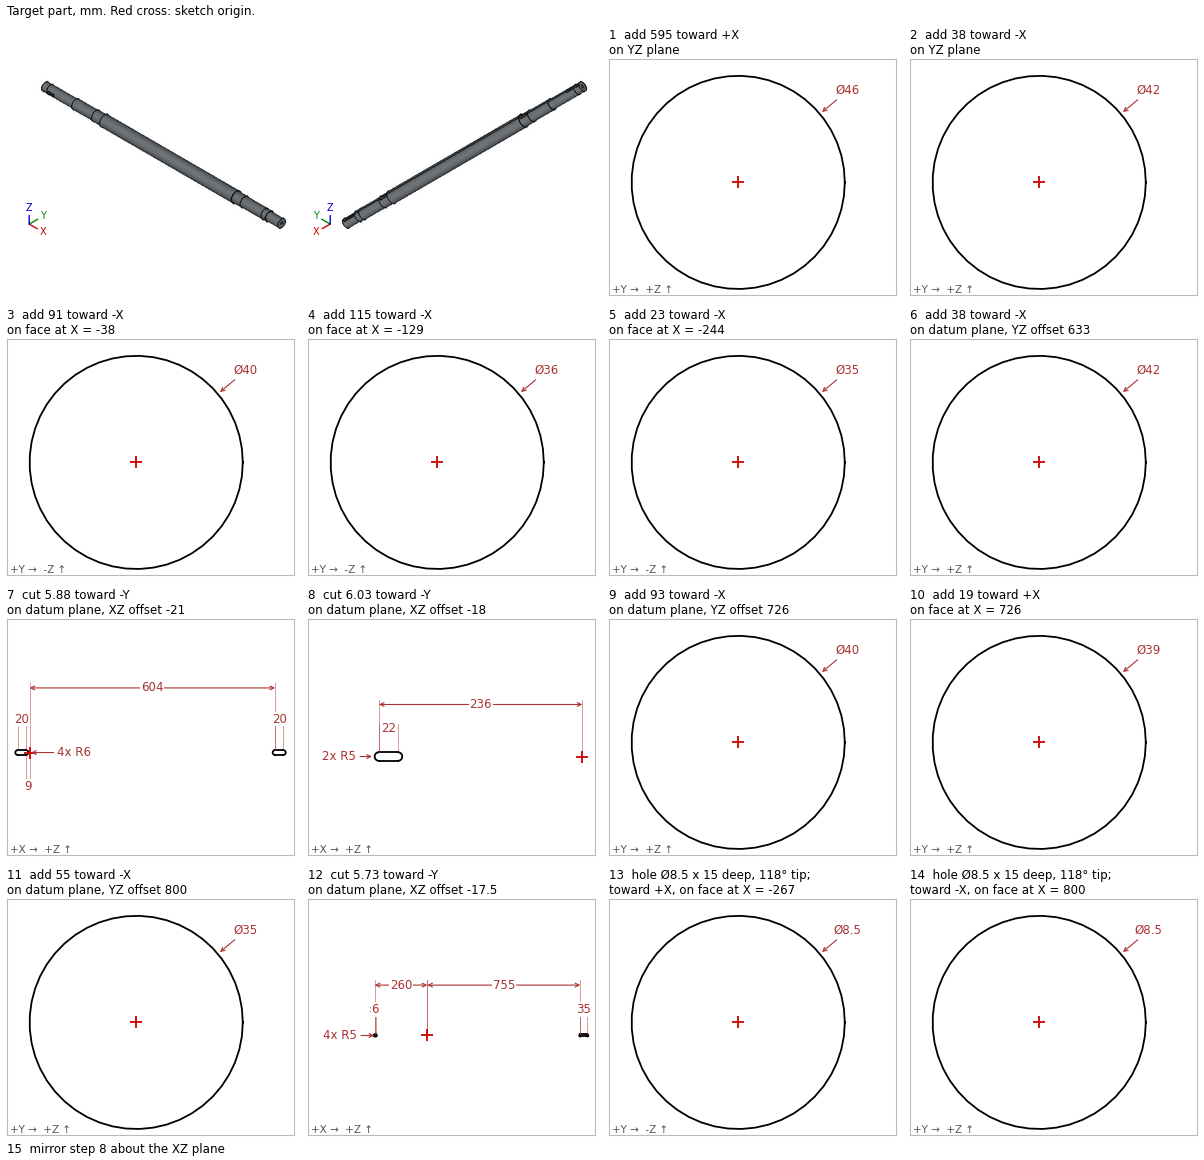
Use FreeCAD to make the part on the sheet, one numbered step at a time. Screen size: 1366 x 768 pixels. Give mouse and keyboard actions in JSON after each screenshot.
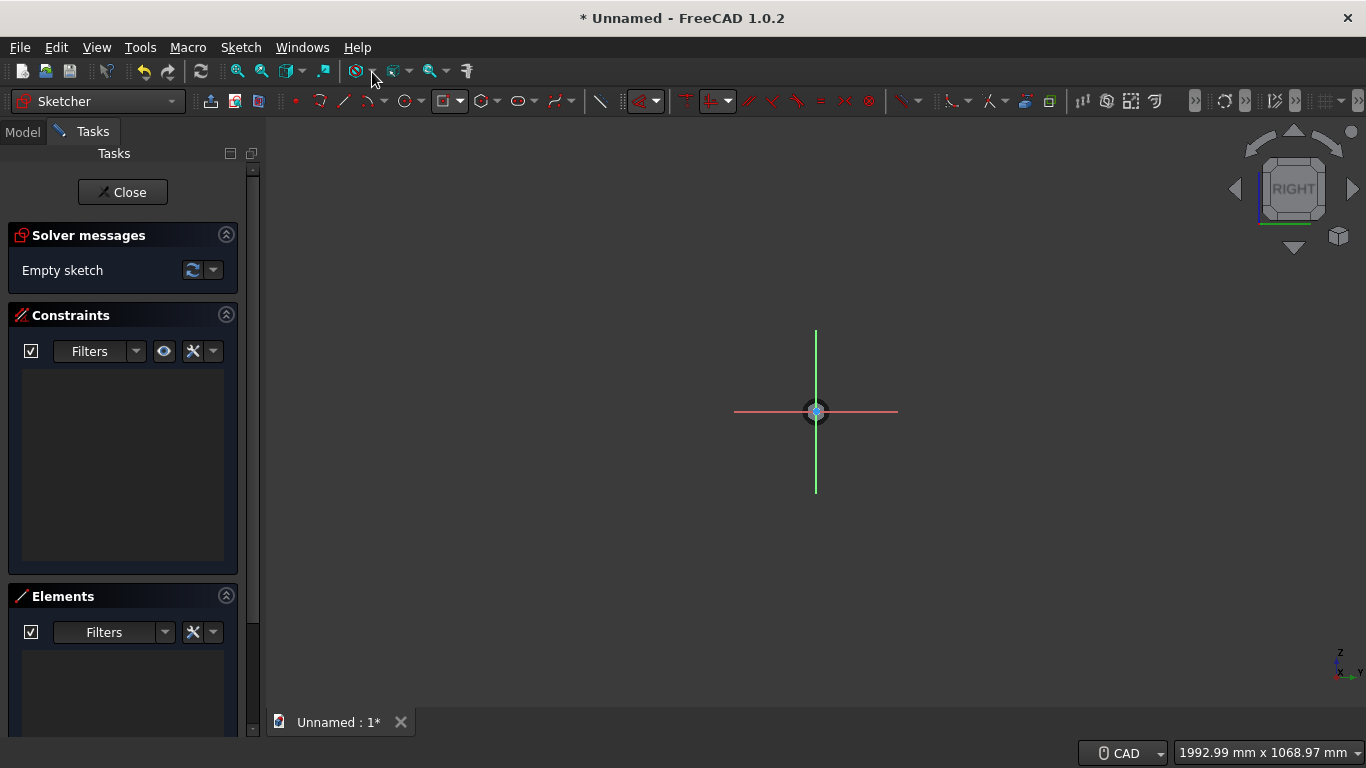
{"action": "scroll", "coordinate": [820, 412], "scroll_direction": "up", "scroll_amount": 15}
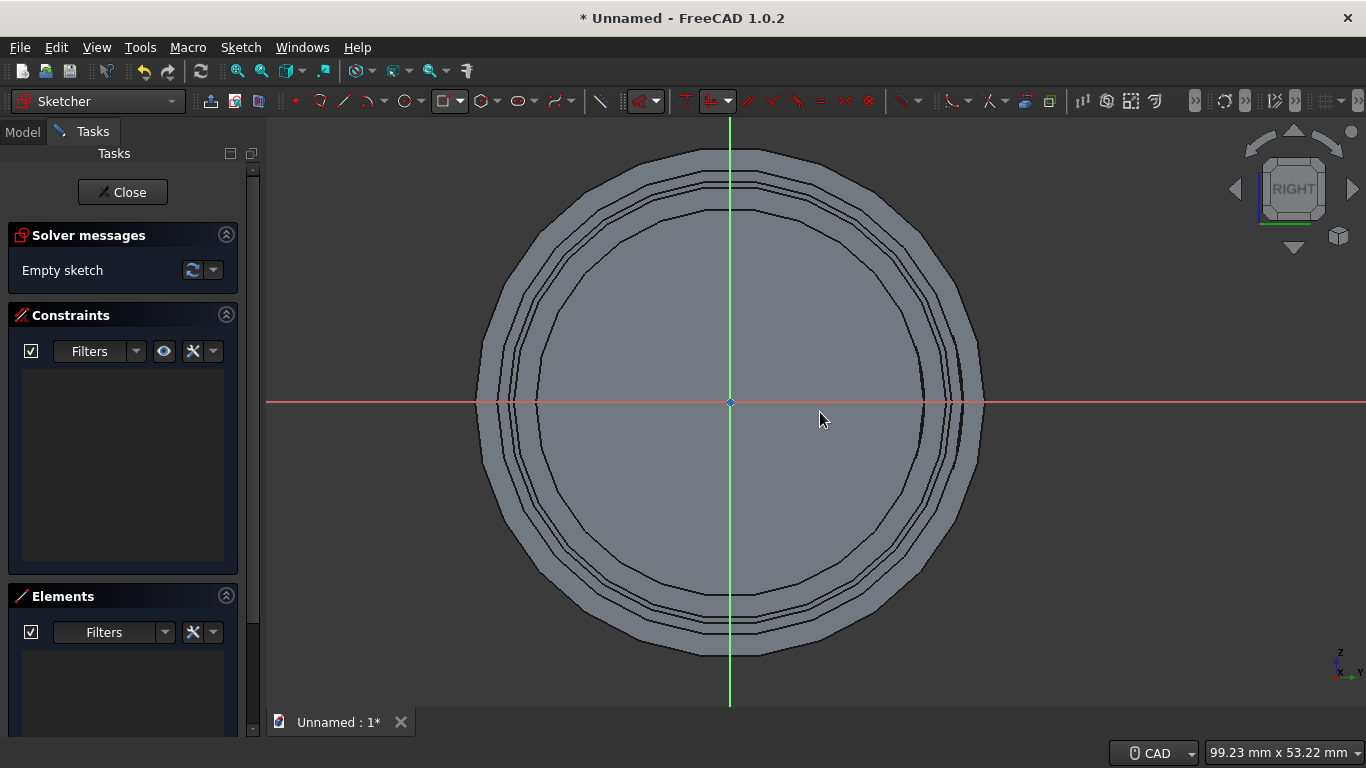
{"action": "scroll", "coordinate": [724, 399], "scroll_direction": "up", "scroll_amount": 7}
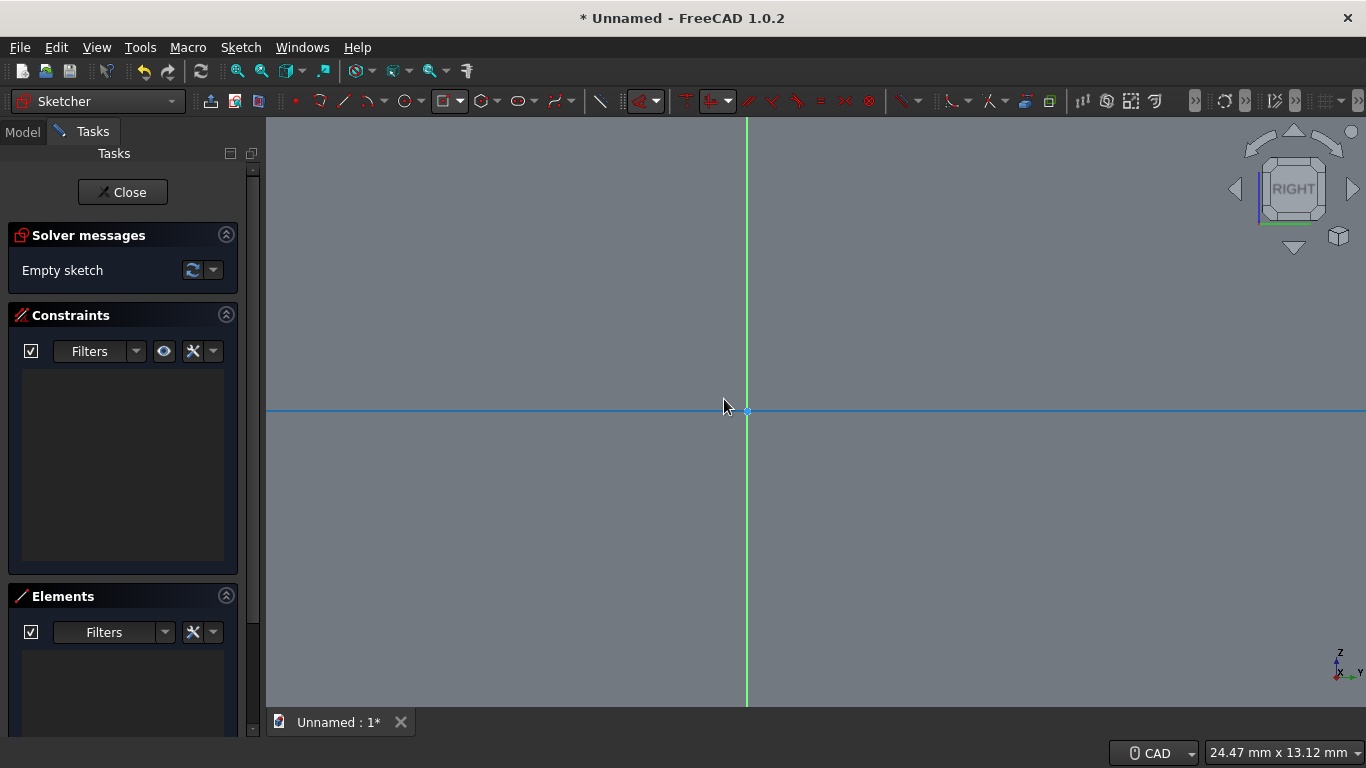
{"action": "left_click", "coordinate": [406, 102]}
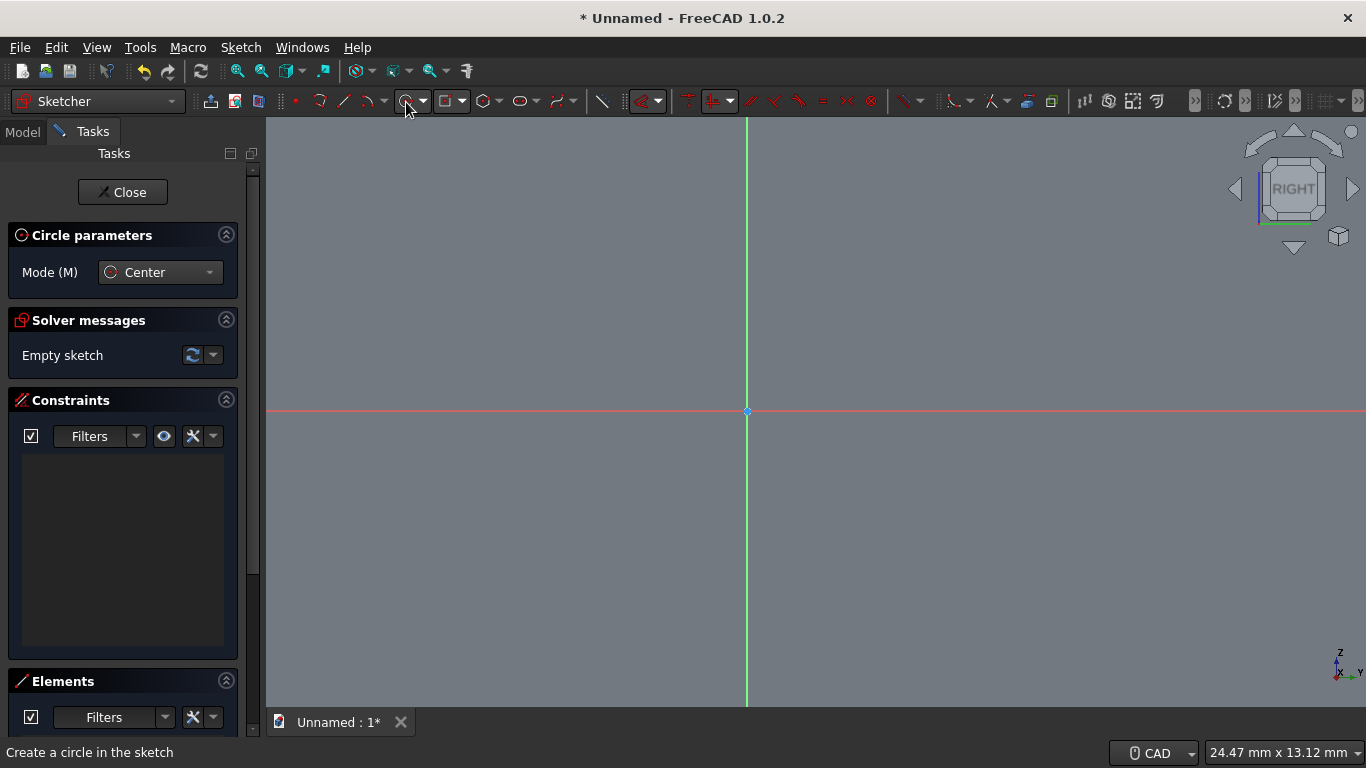
{"action": "left_click", "coordinate": [747, 411]}
{"action": "mouse_move", "coordinate": [882, 276]}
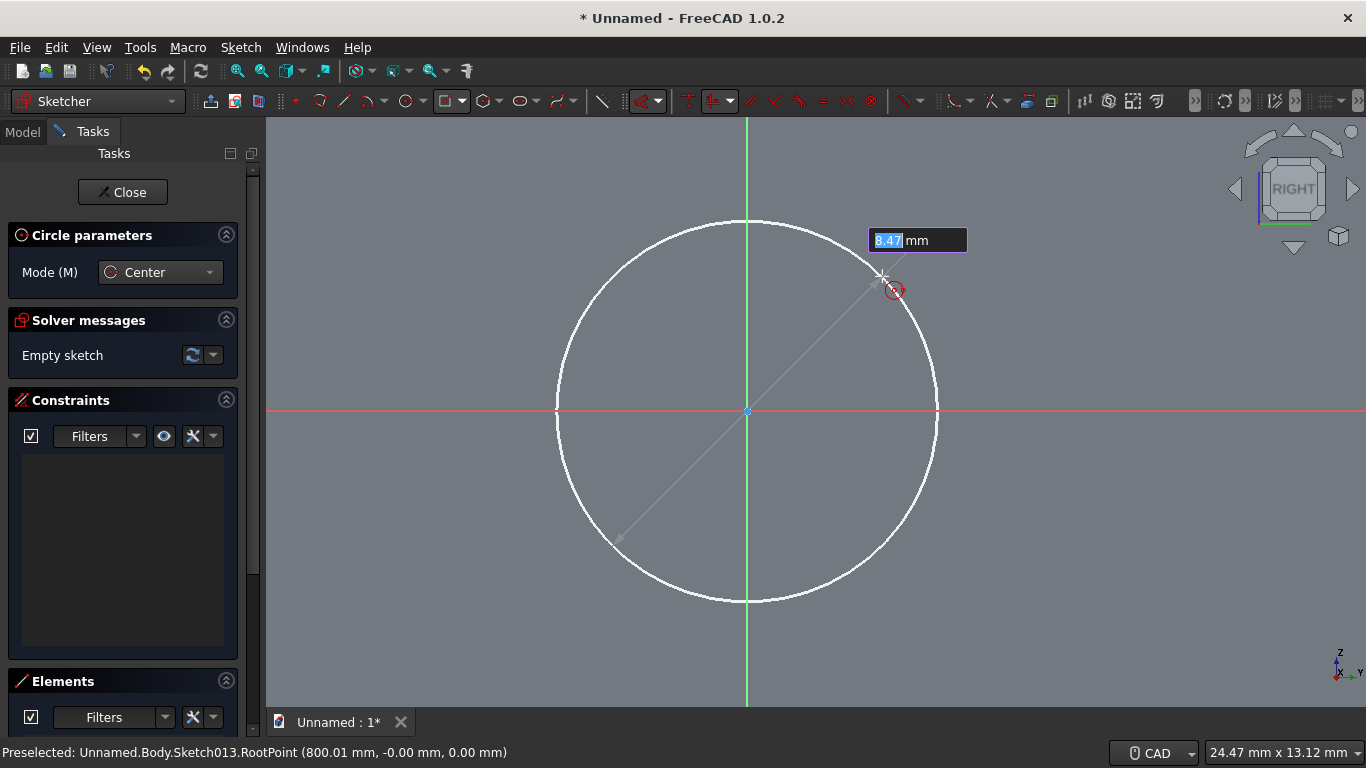
{"action": "type", "text": "8.5"}
{"action": "key", "text": "Return"}
{"action": "key", "text": "Escape"}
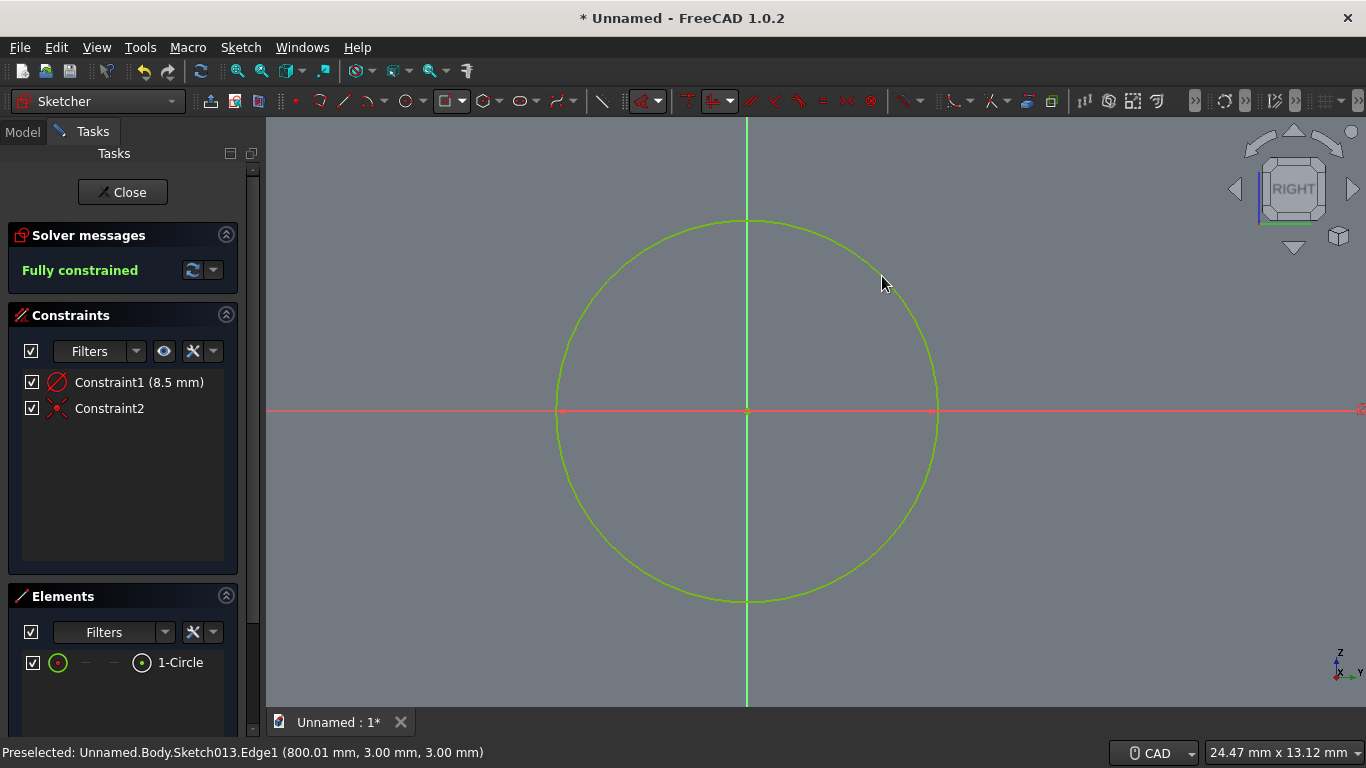
{"action": "left_click", "coordinate": [123, 192]}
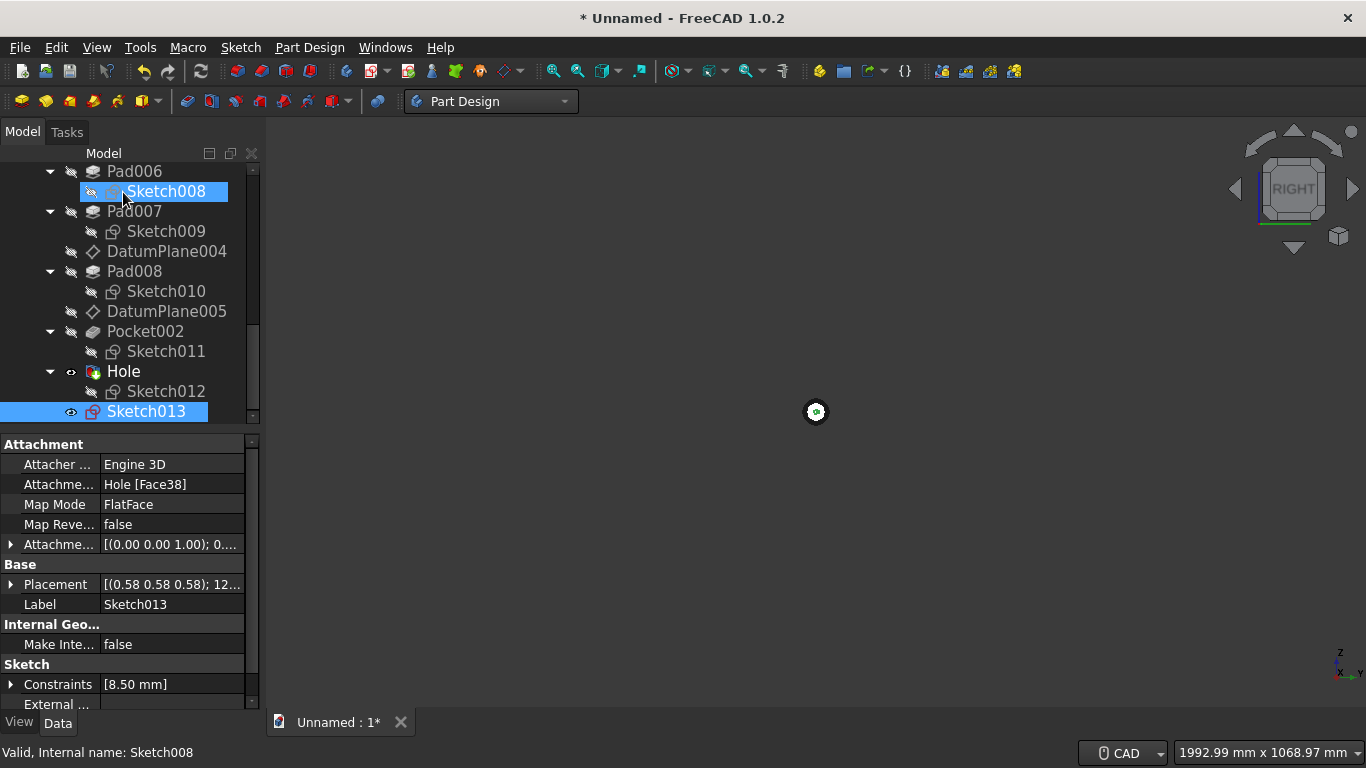
{"action": "left_click", "coordinate": [212, 102]}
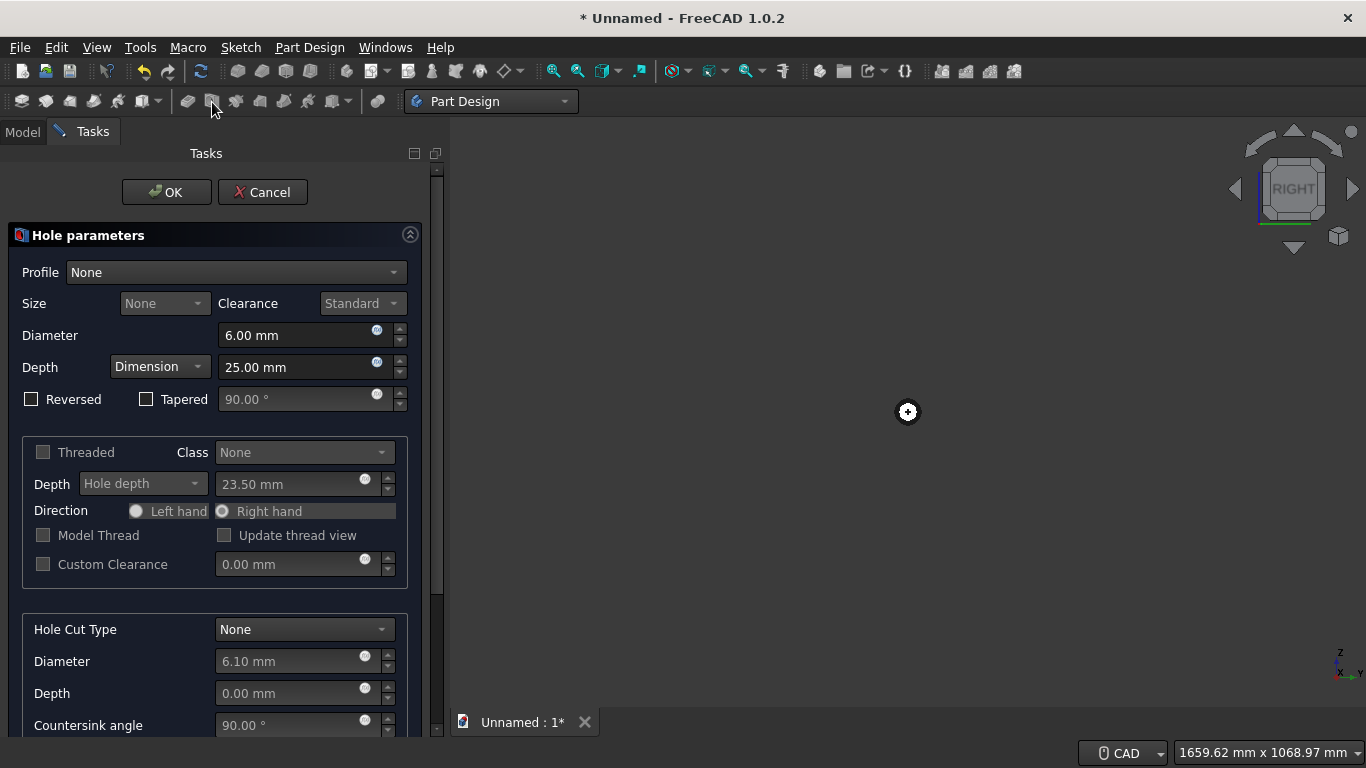
{"action": "triple_click", "coordinate": [305, 335]}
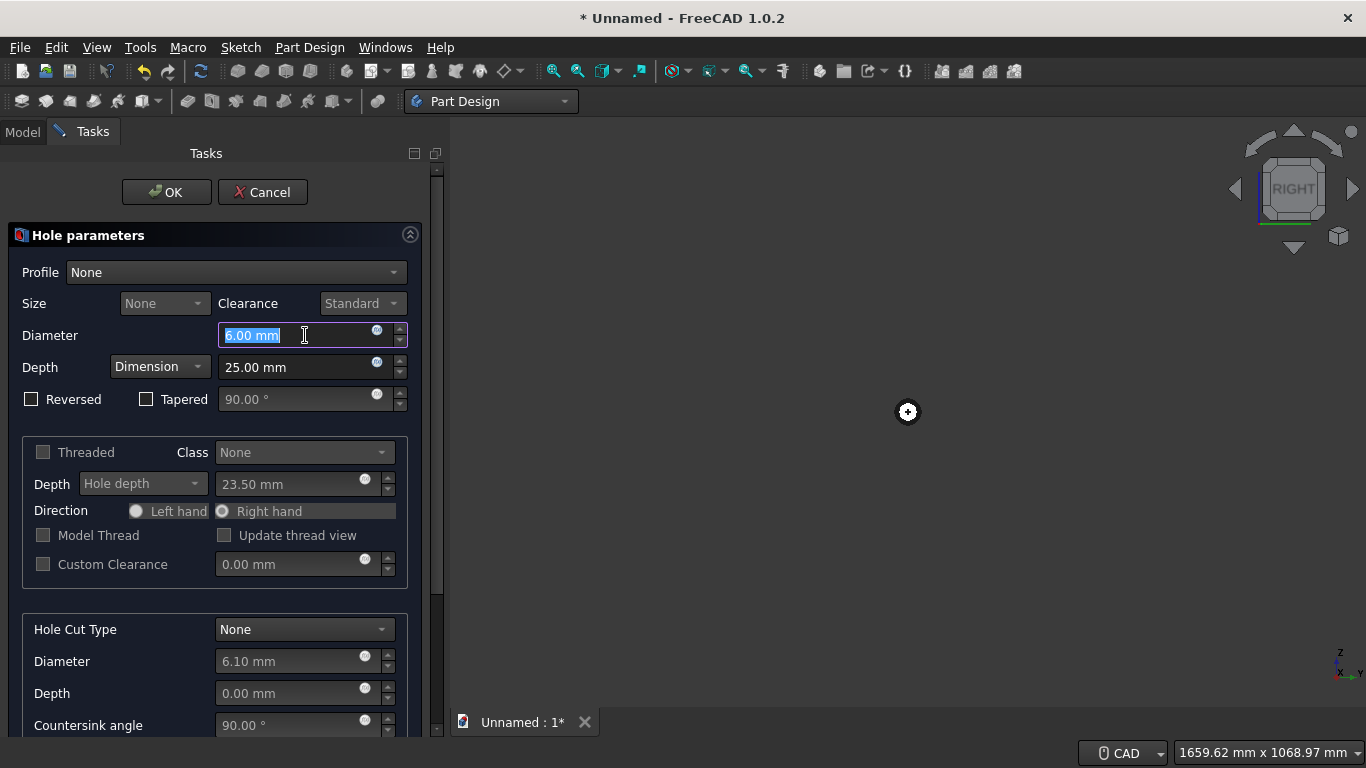
{"action": "type", "text": "8.5"}
{"action": "key", "text": "Tab"}